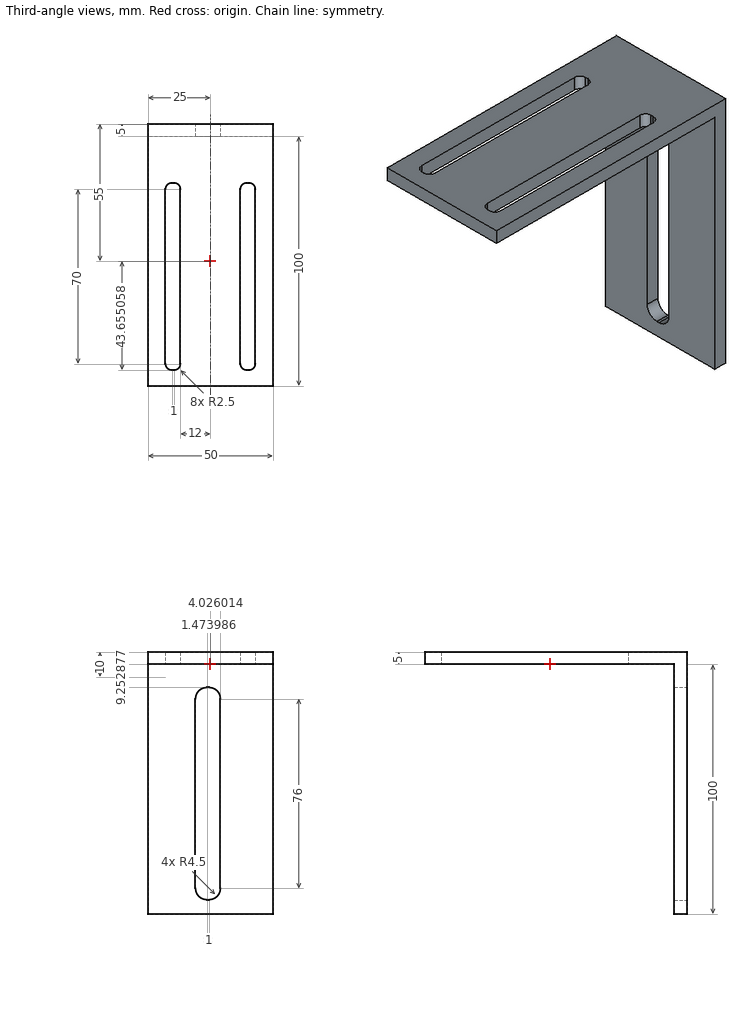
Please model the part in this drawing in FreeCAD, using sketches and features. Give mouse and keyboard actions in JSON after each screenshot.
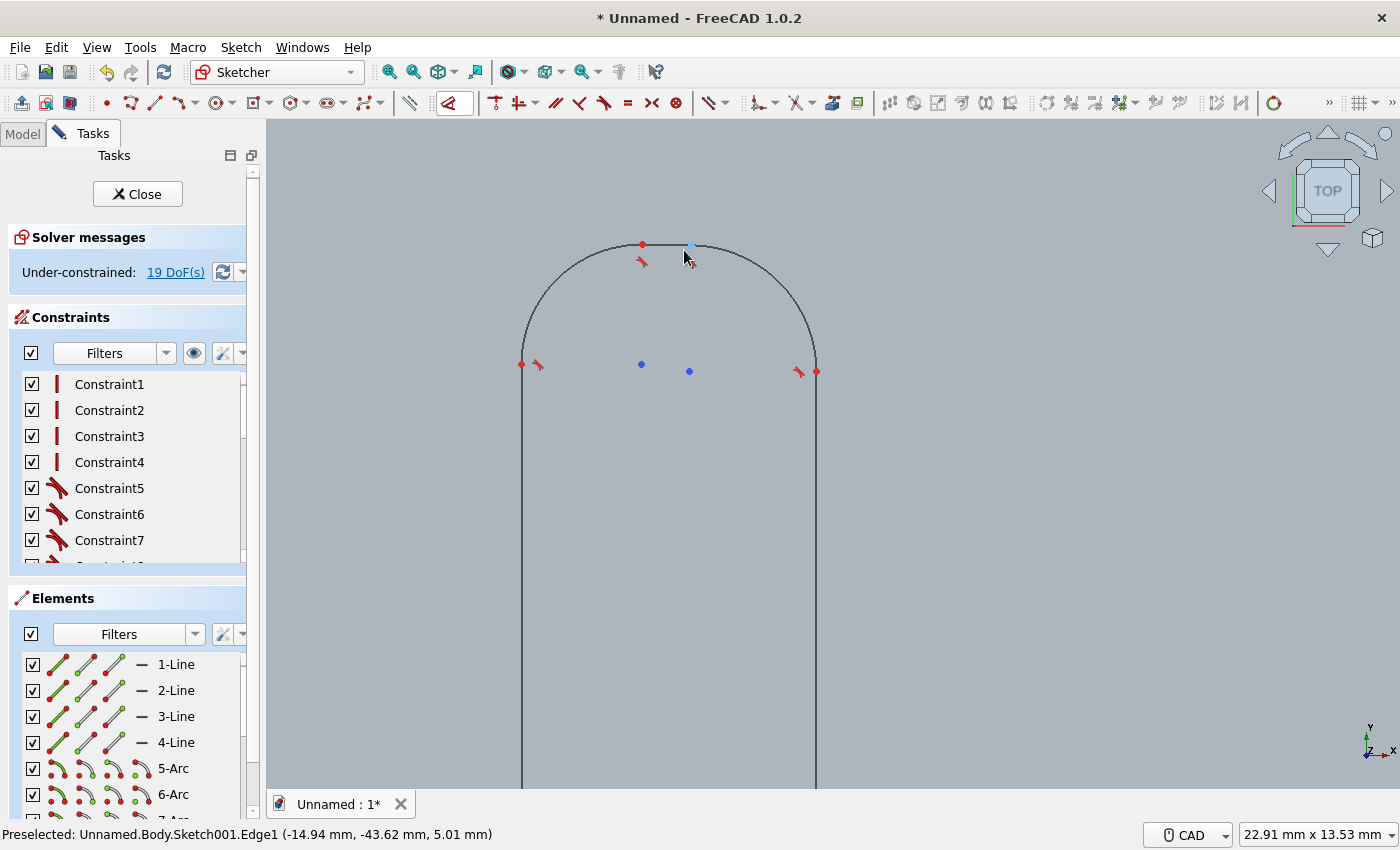
{"action": "left_click", "coordinate": [677, 245]}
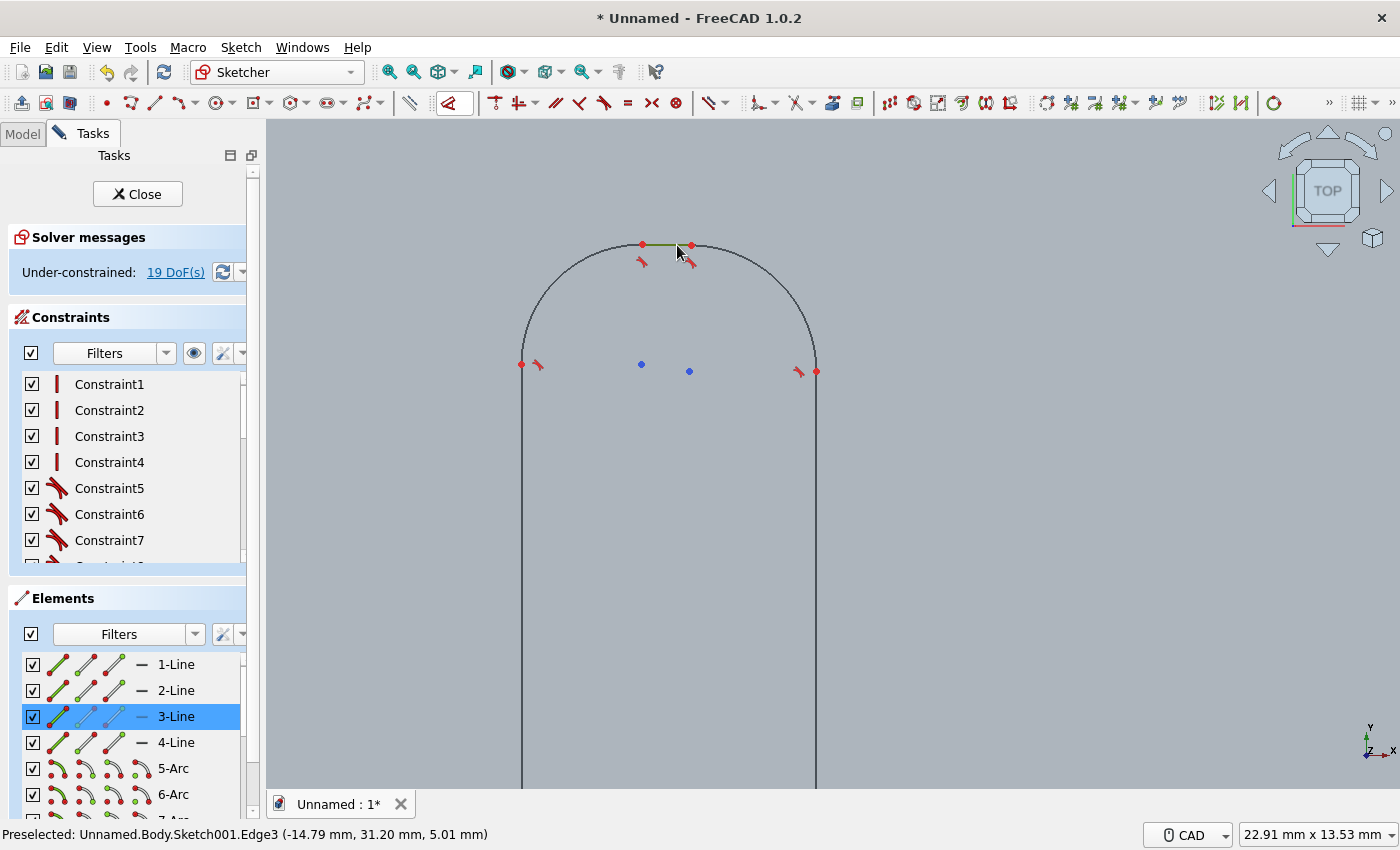
{"action": "key", "text": "h"}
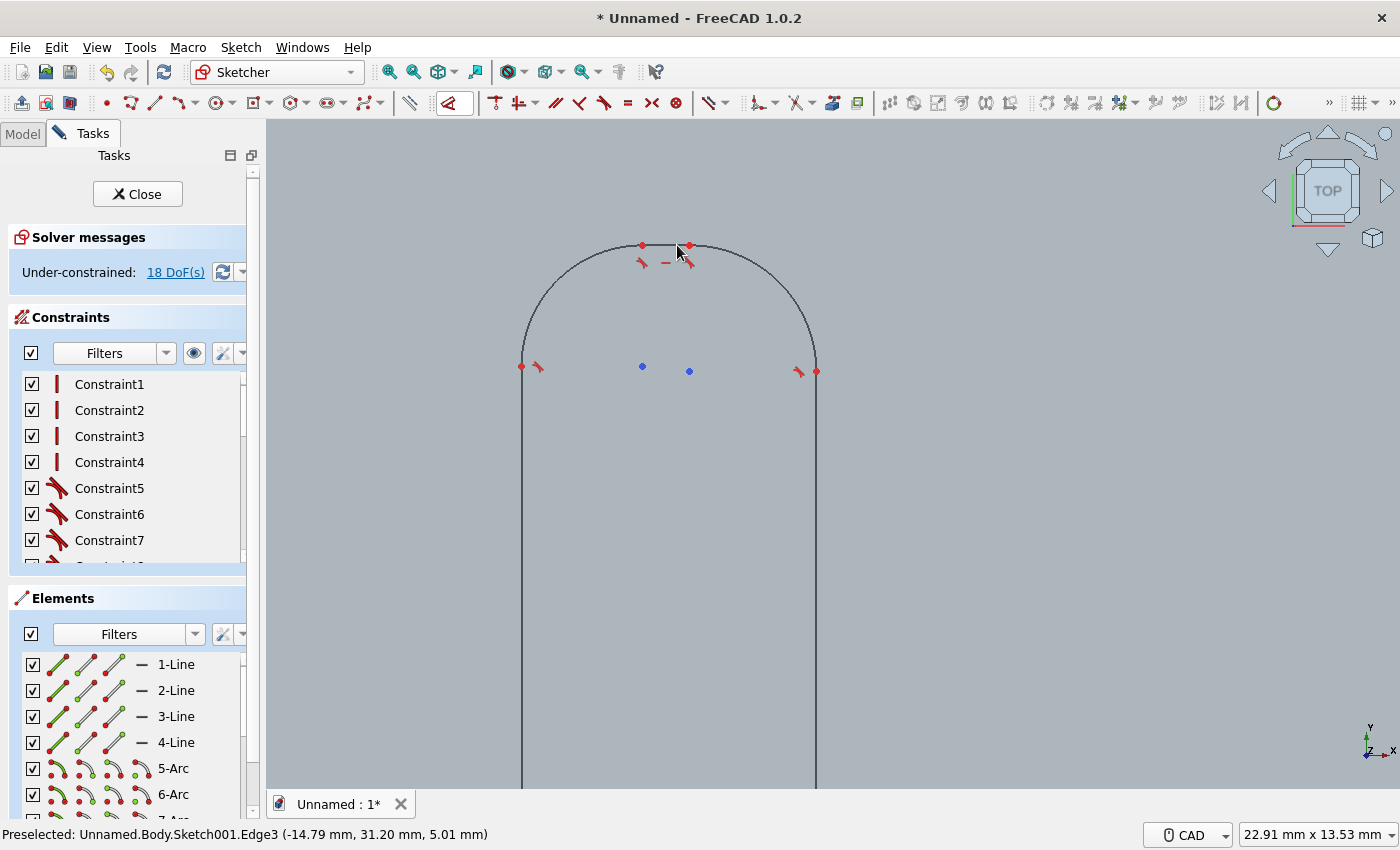
{"action": "scroll", "coordinate": [684, 250], "scroll_direction": "down", "scroll_amount": 11}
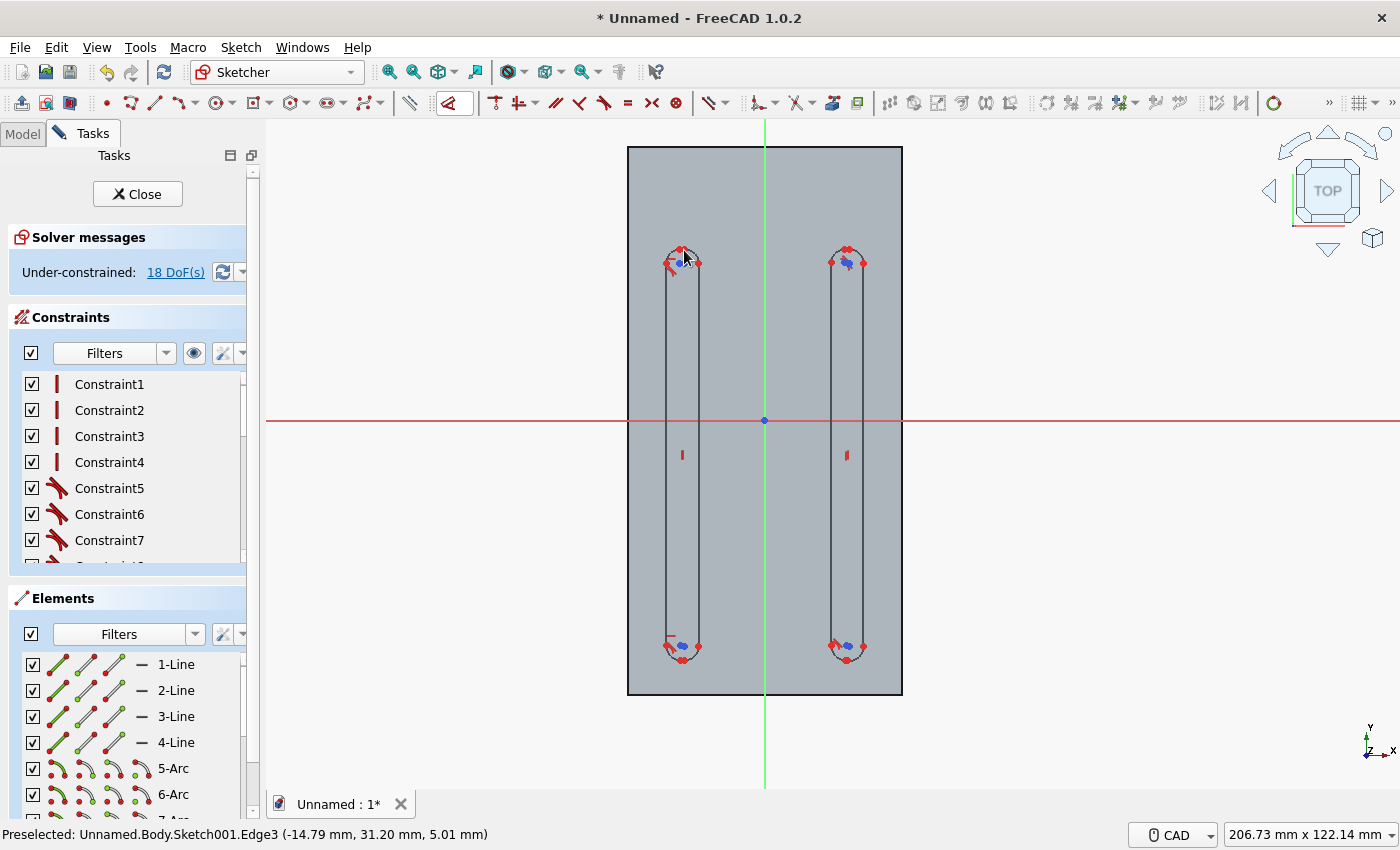
{"action": "scroll", "coordinate": [846, 661], "scroll_direction": "up", "scroll_amount": 13}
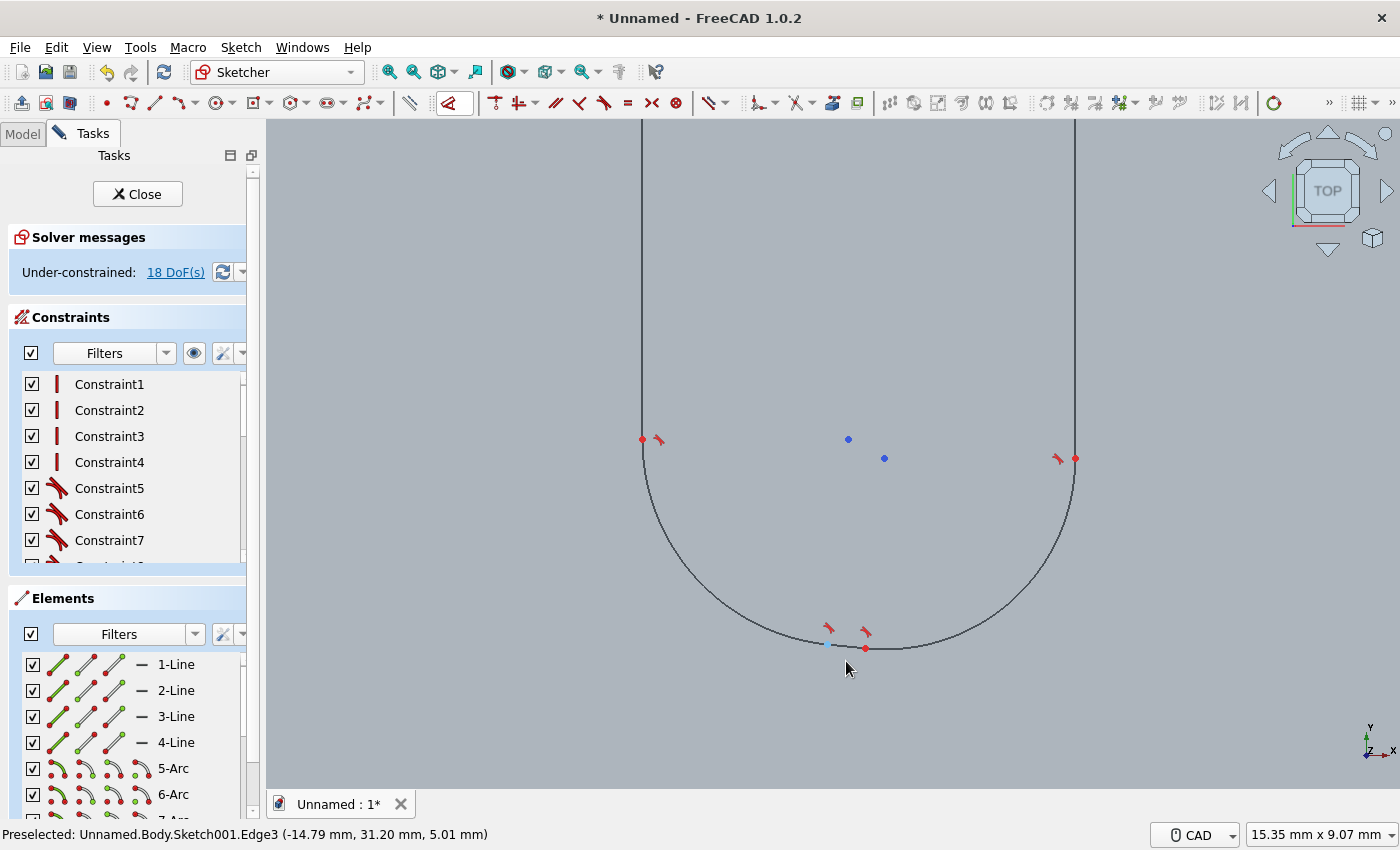
{"action": "left_click", "coordinate": [843, 646]}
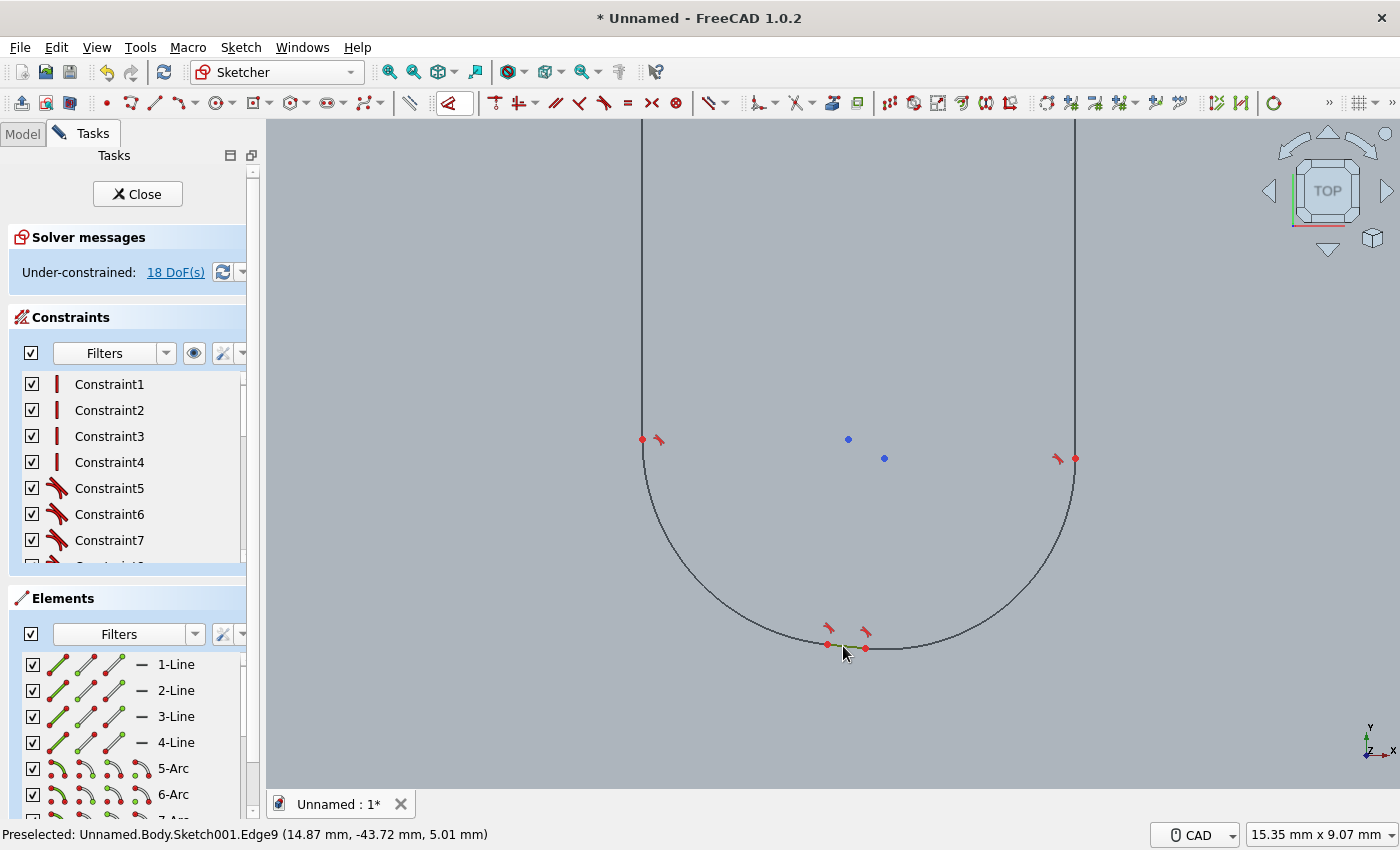
{"action": "key", "text": "h"}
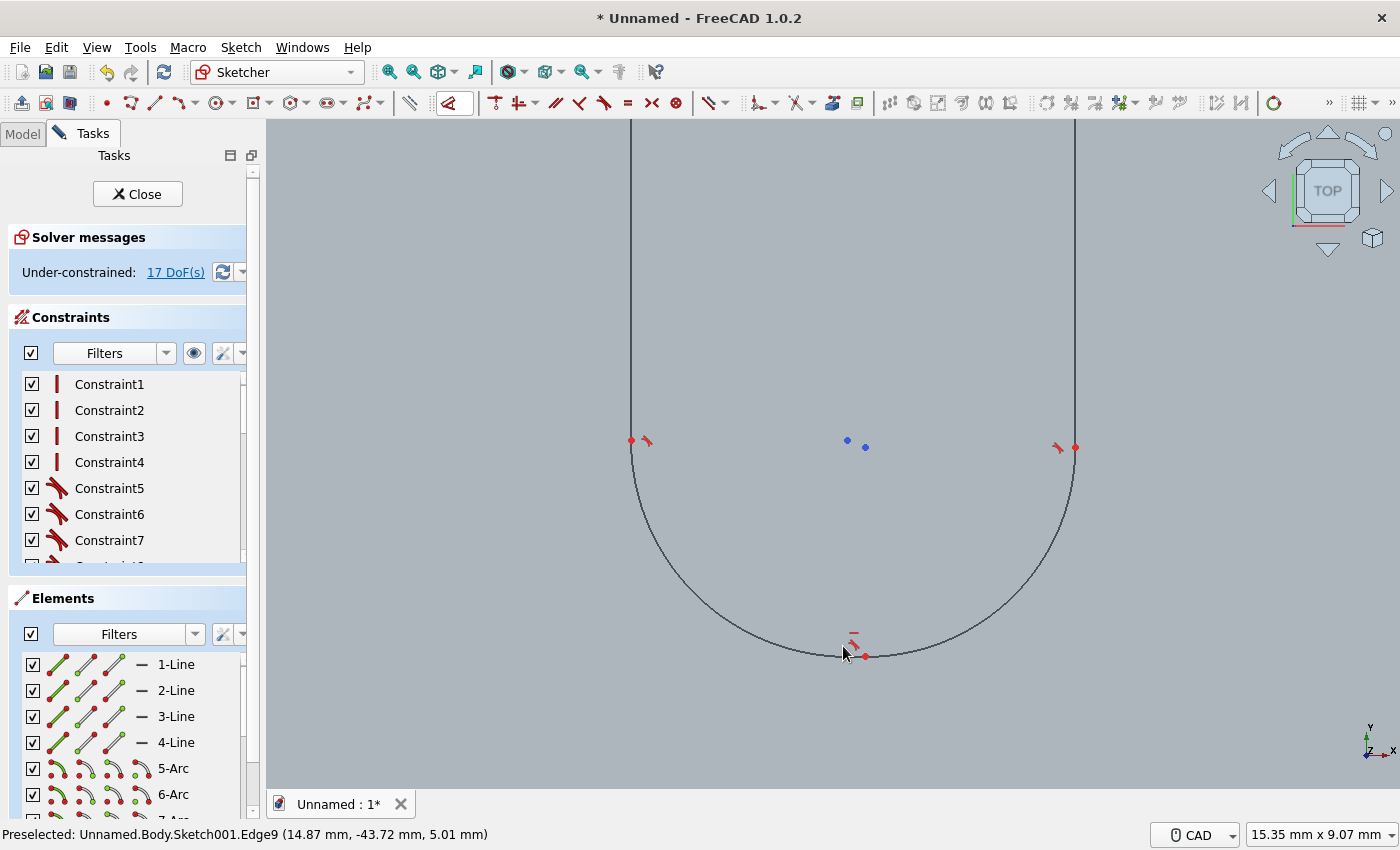
{"action": "scroll", "coordinate": [846, 661], "scroll_direction": "down", "scroll_amount": 13}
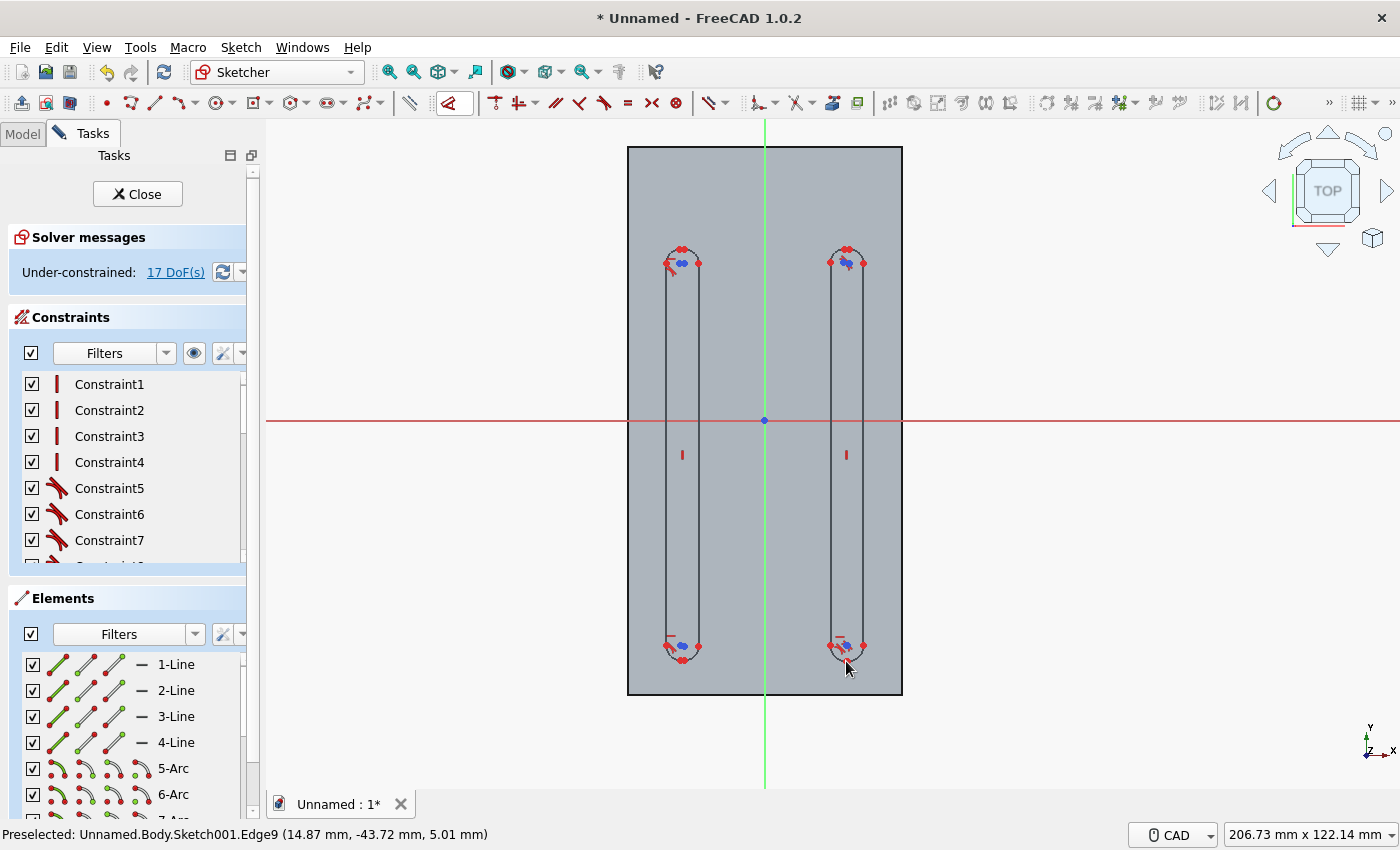
{"action": "scroll", "coordinate": [848, 249], "scroll_direction": "up", "scroll_amount": 11}